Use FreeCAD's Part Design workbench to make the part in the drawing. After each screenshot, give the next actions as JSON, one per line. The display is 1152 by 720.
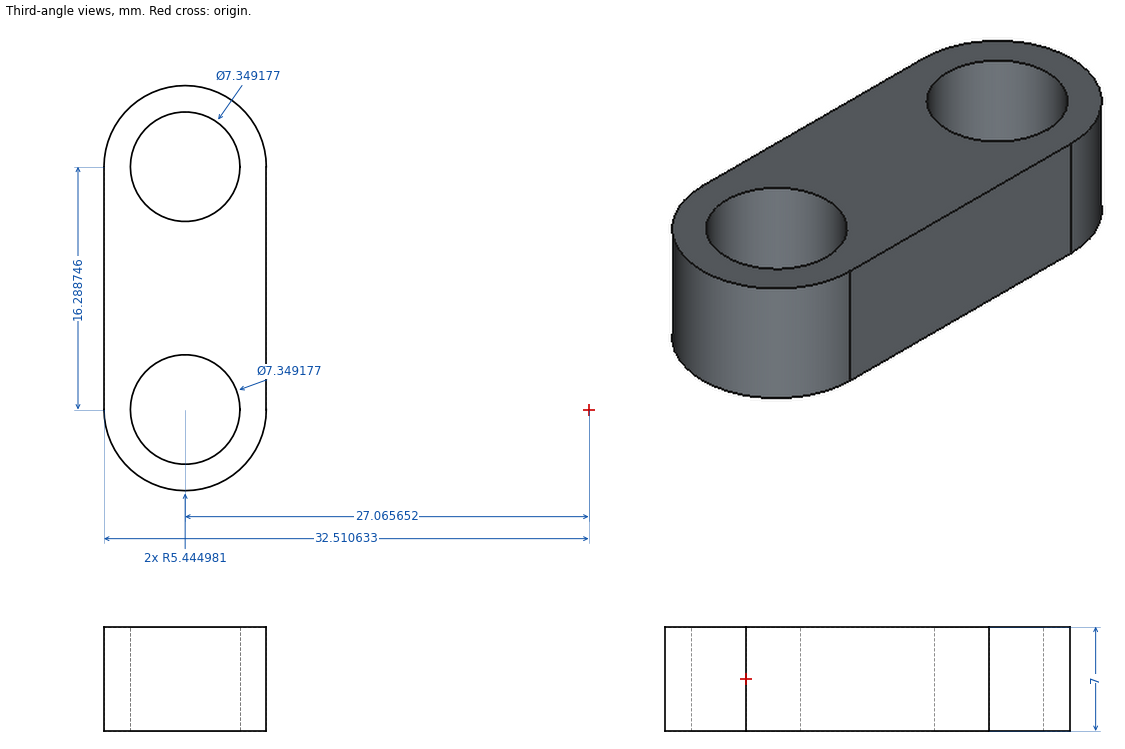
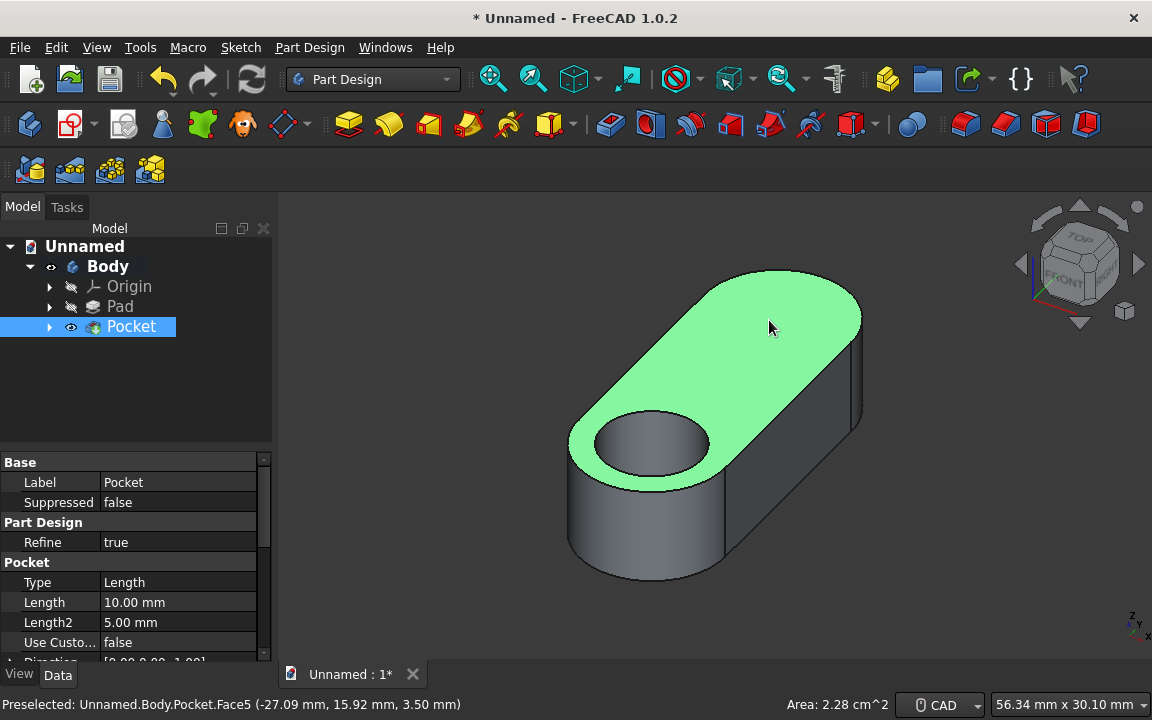
{"action": "left_click", "coordinate": [70, 124]}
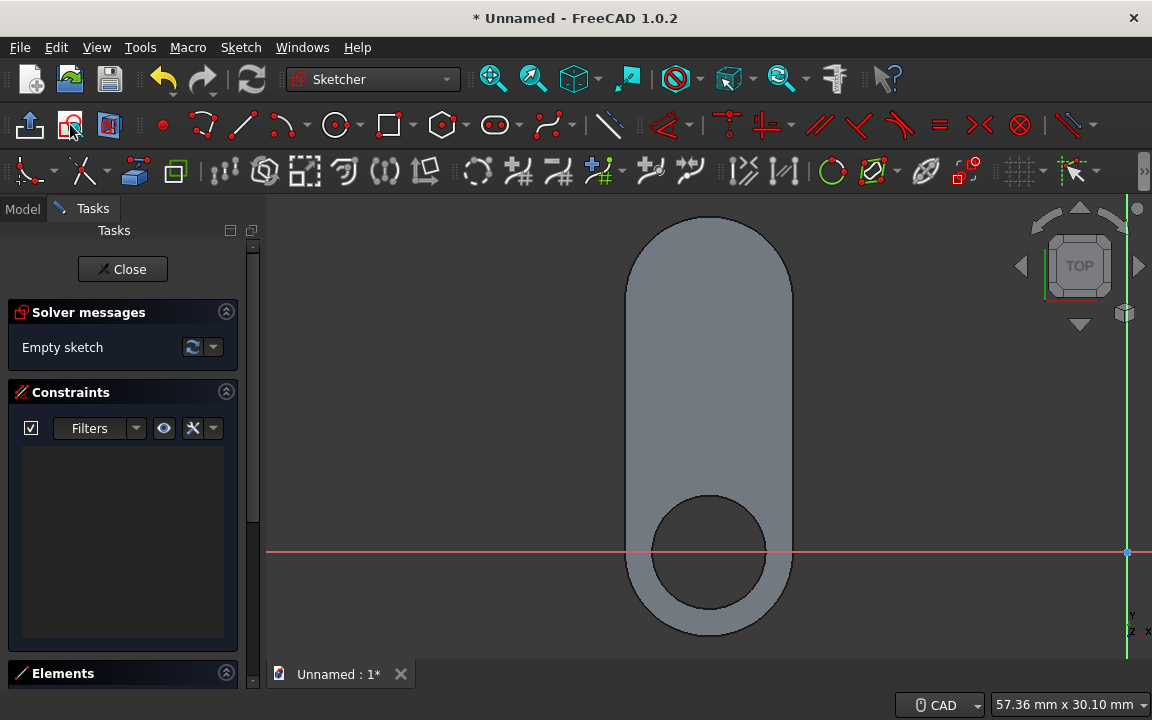
{"action": "scroll", "coordinate": [749, 227], "scroll_direction": "up", "scroll_amount": 5}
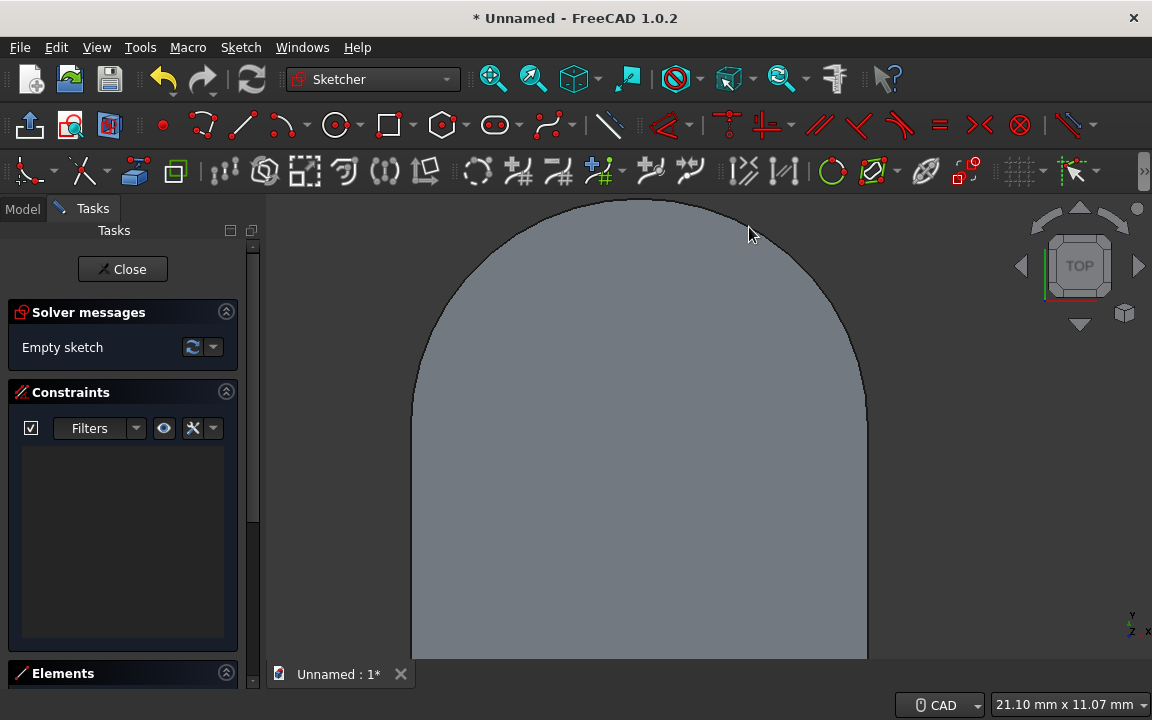
{"action": "left_click", "coordinate": [336, 126]}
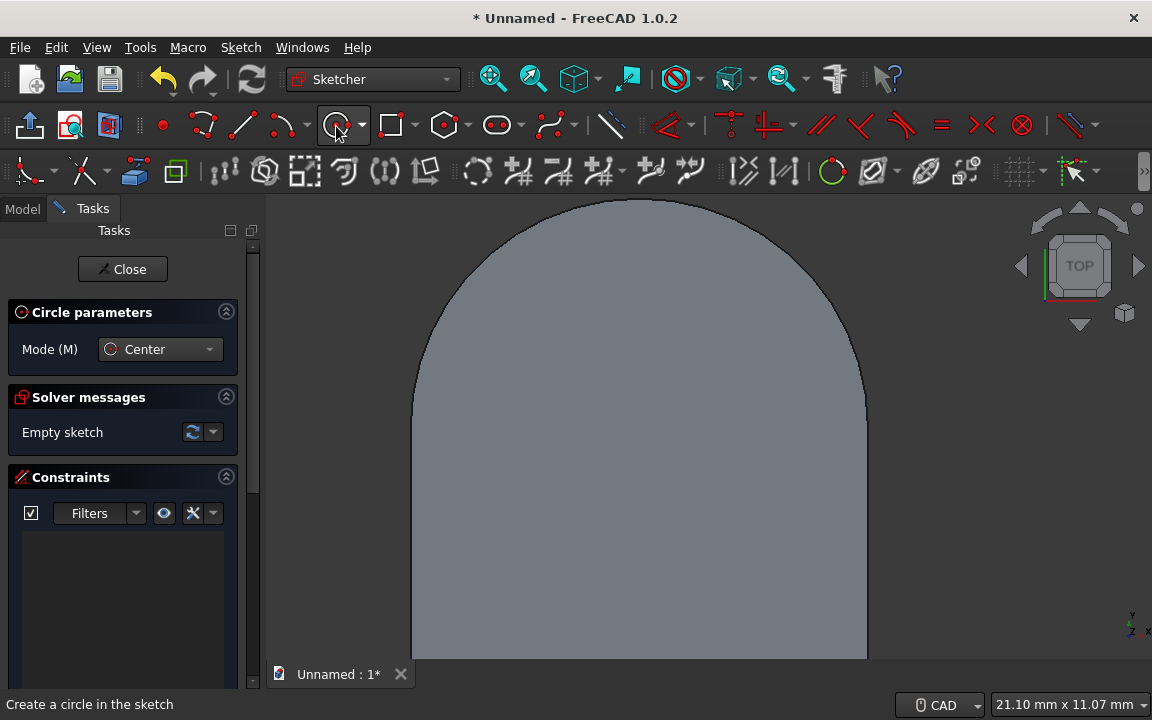
{"action": "left_click", "coordinate": [639, 427]}
{"action": "mouse_move", "coordinate": [748, 318]}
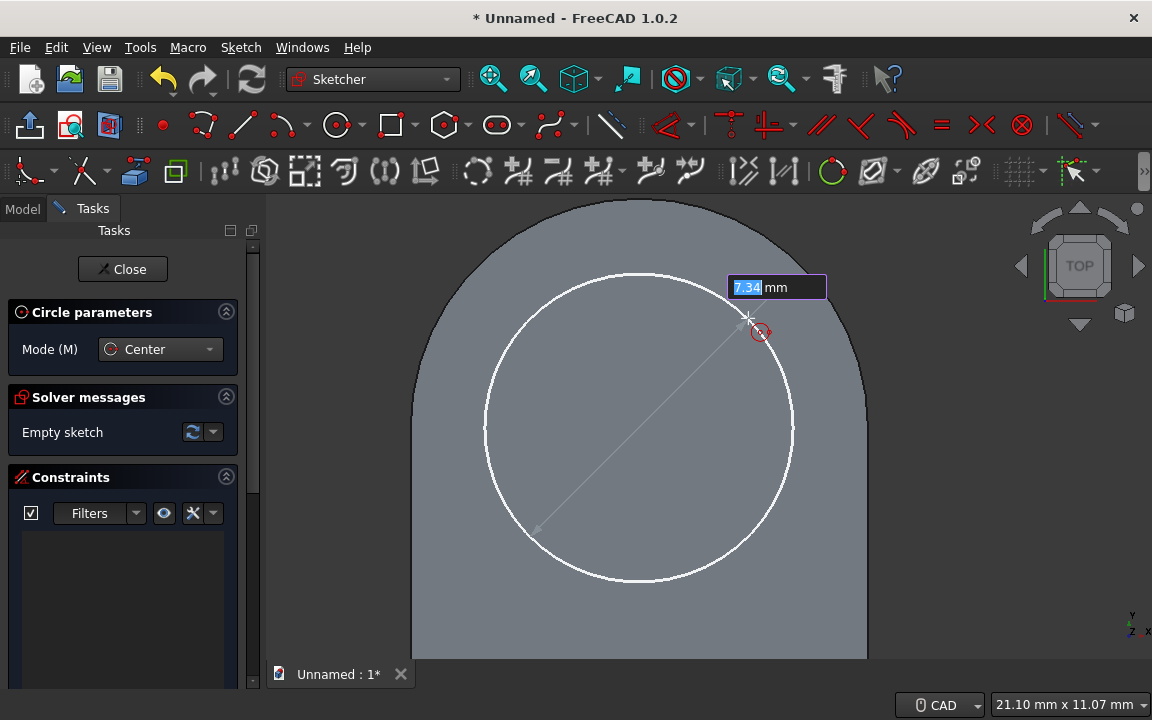
{"action": "type", "text": "7.349177"}
{"action": "key", "text": "Return"}
{"action": "key", "text": "Escape"}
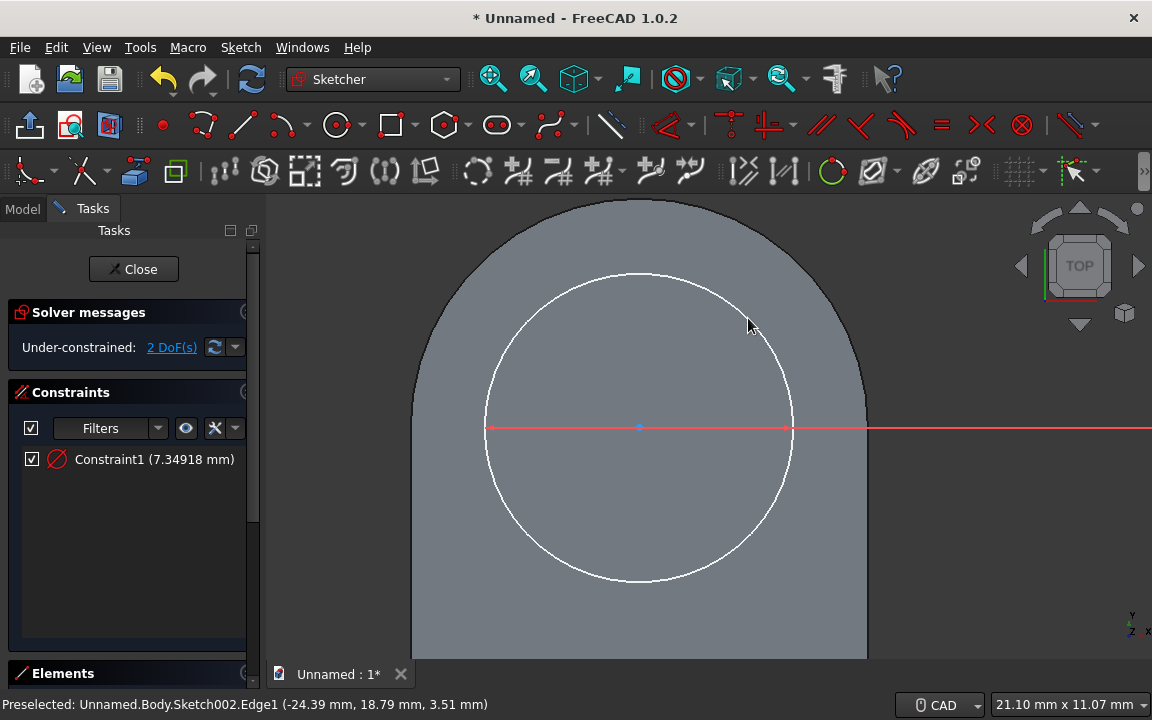
{"action": "left_click", "coordinate": [666, 126]}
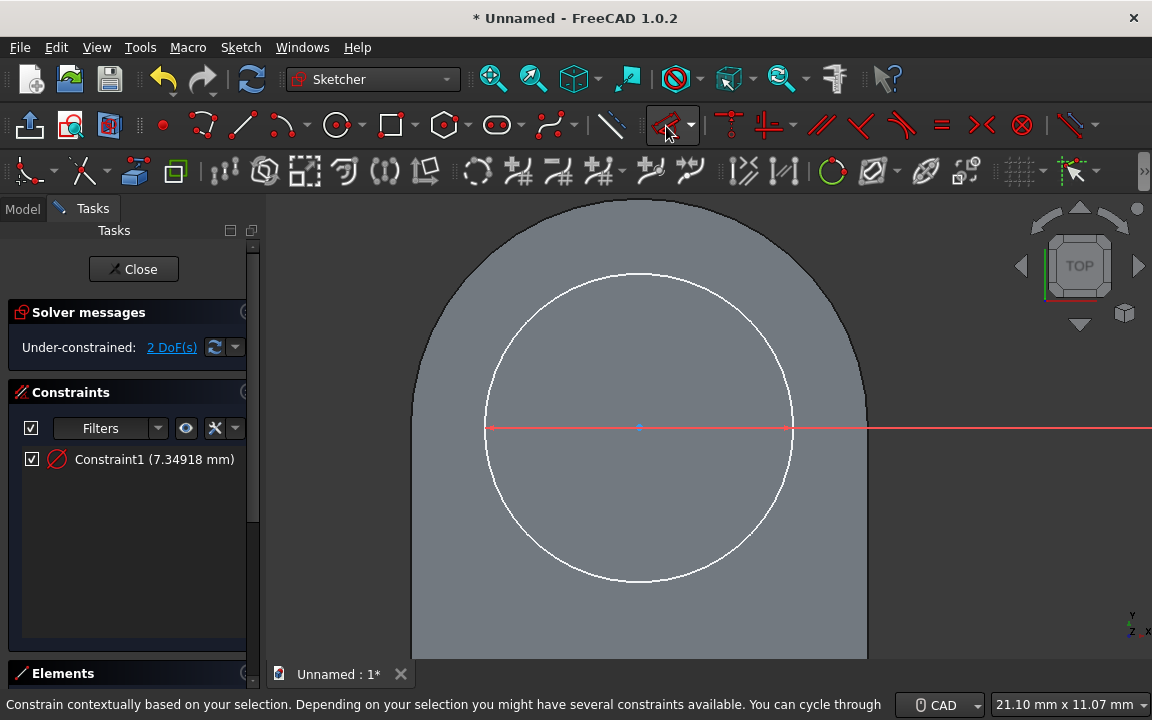
{"action": "left_click", "coordinate": [639, 428]}
{"action": "left_click", "coordinate": [813, 394]}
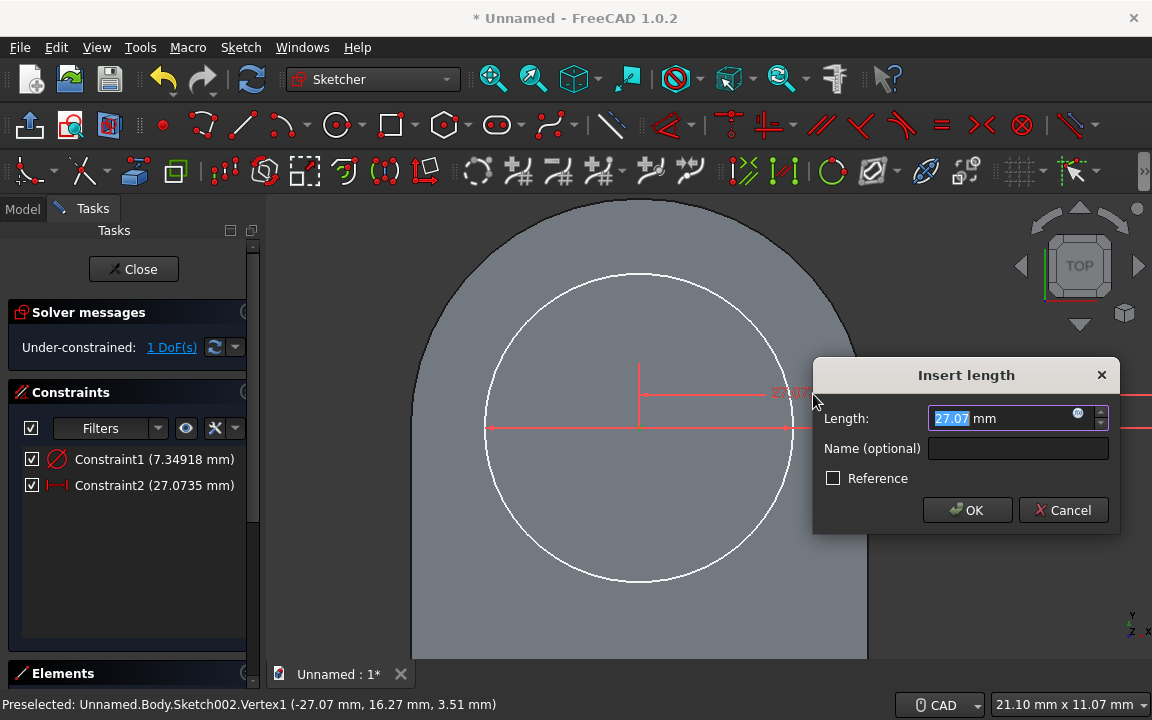
{"action": "type", "text": "27.065652"}
{"action": "key", "text": "Return"}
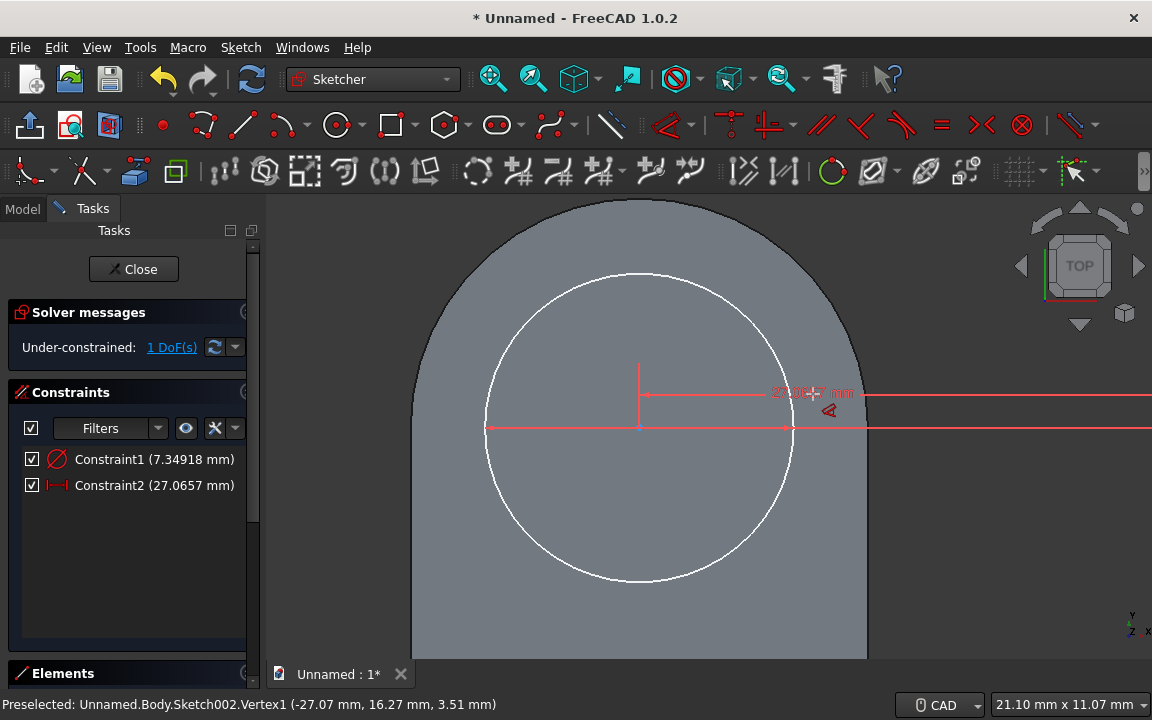
{"action": "left_click", "coordinate": [639, 428]}
{"action": "left_click", "coordinate": [605, 529]}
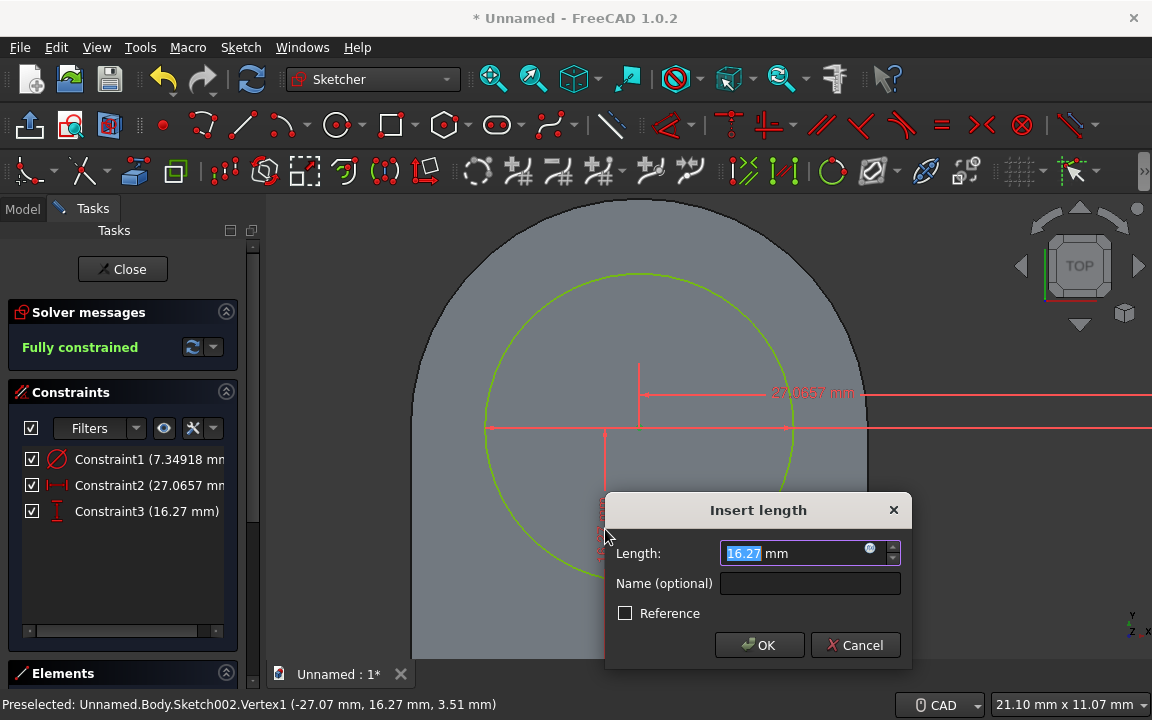
{"action": "type", "text": "16.288746"}
{"action": "key", "text": "Return"}
{"action": "key", "text": "Escape"}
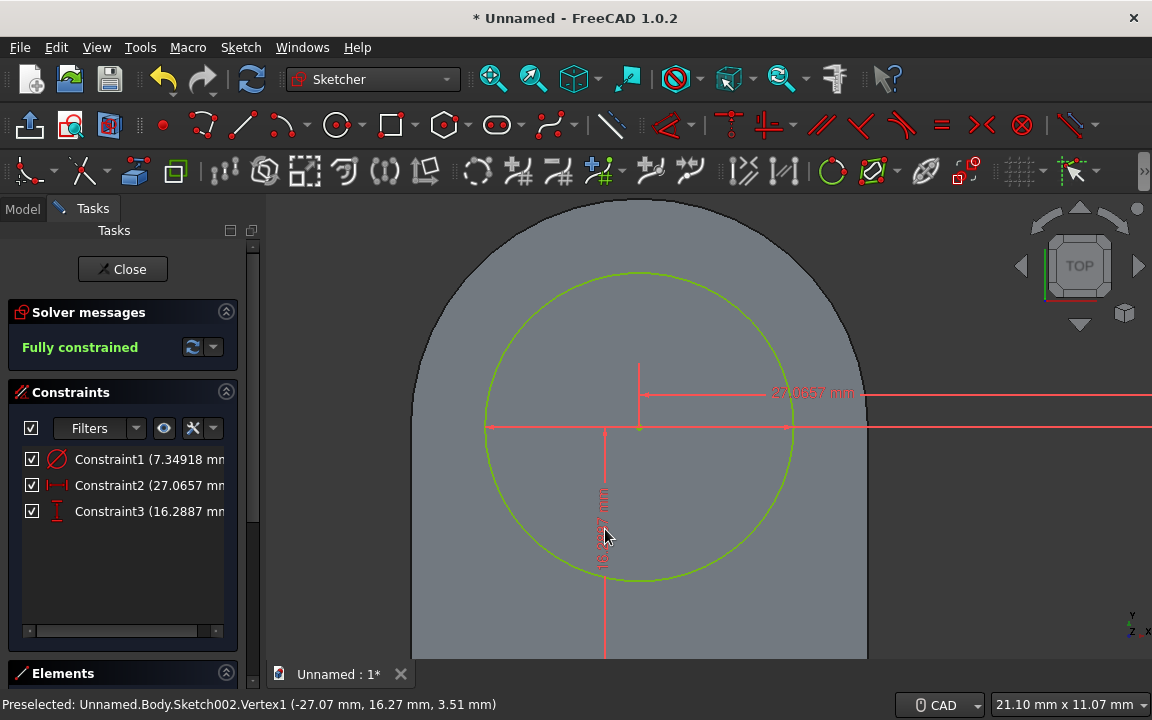
{"action": "left_click", "coordinate": [123, 269]}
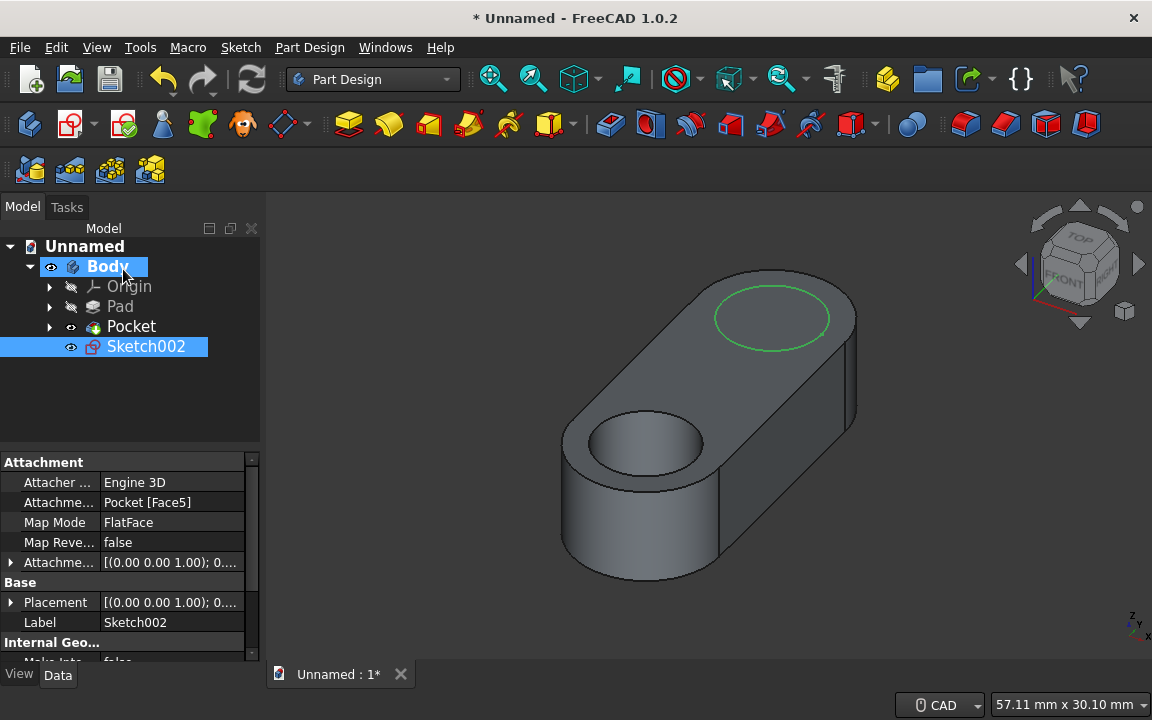
{"action": "left_click", "coordinate": [612, 124]}